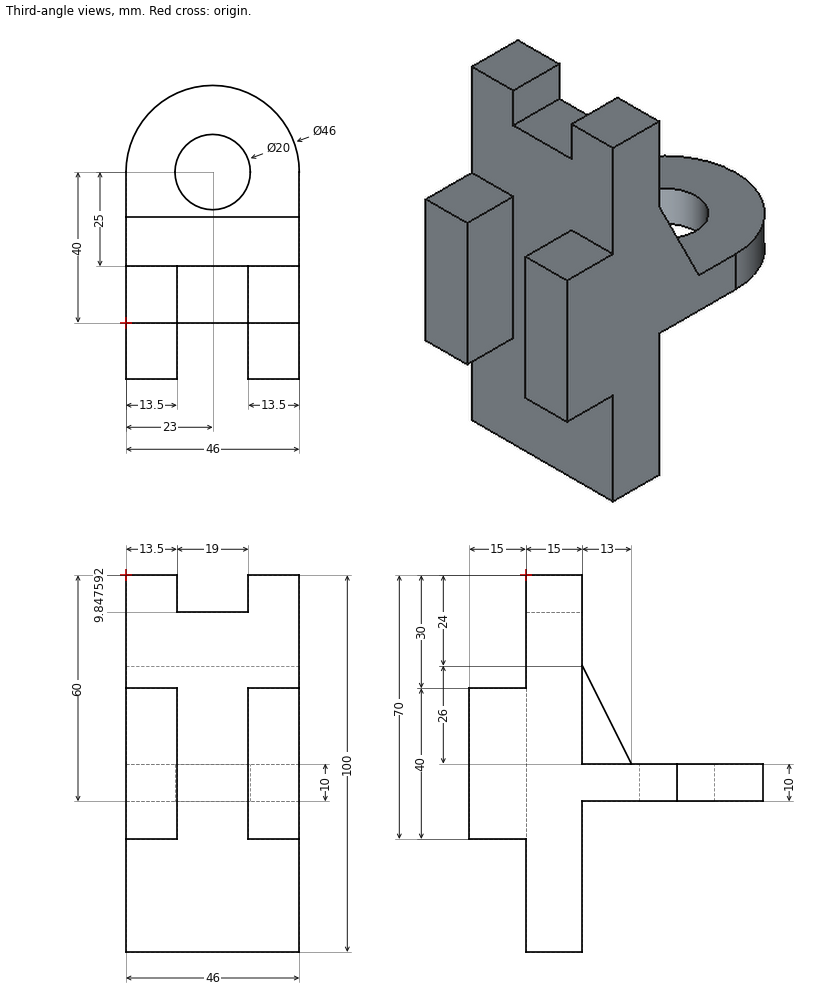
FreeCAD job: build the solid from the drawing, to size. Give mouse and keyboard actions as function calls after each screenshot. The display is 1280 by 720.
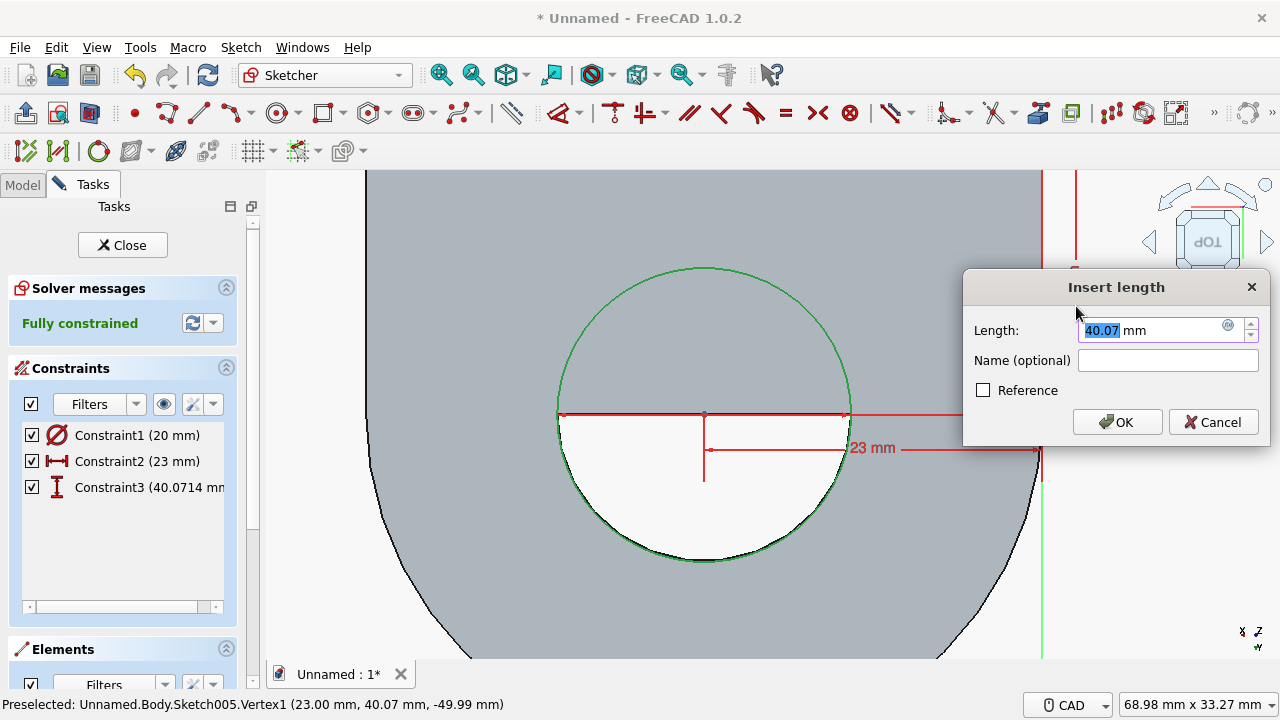
text(40)
key(Return)
key(Escape)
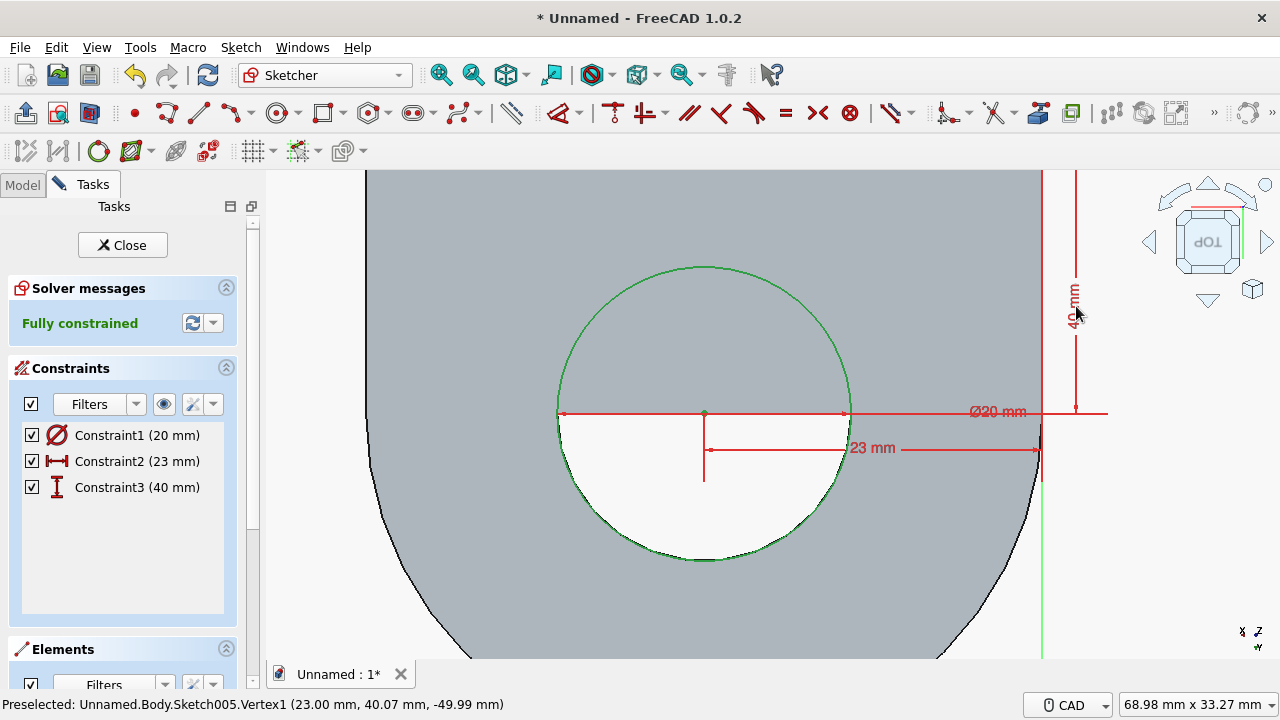
click(123, 245)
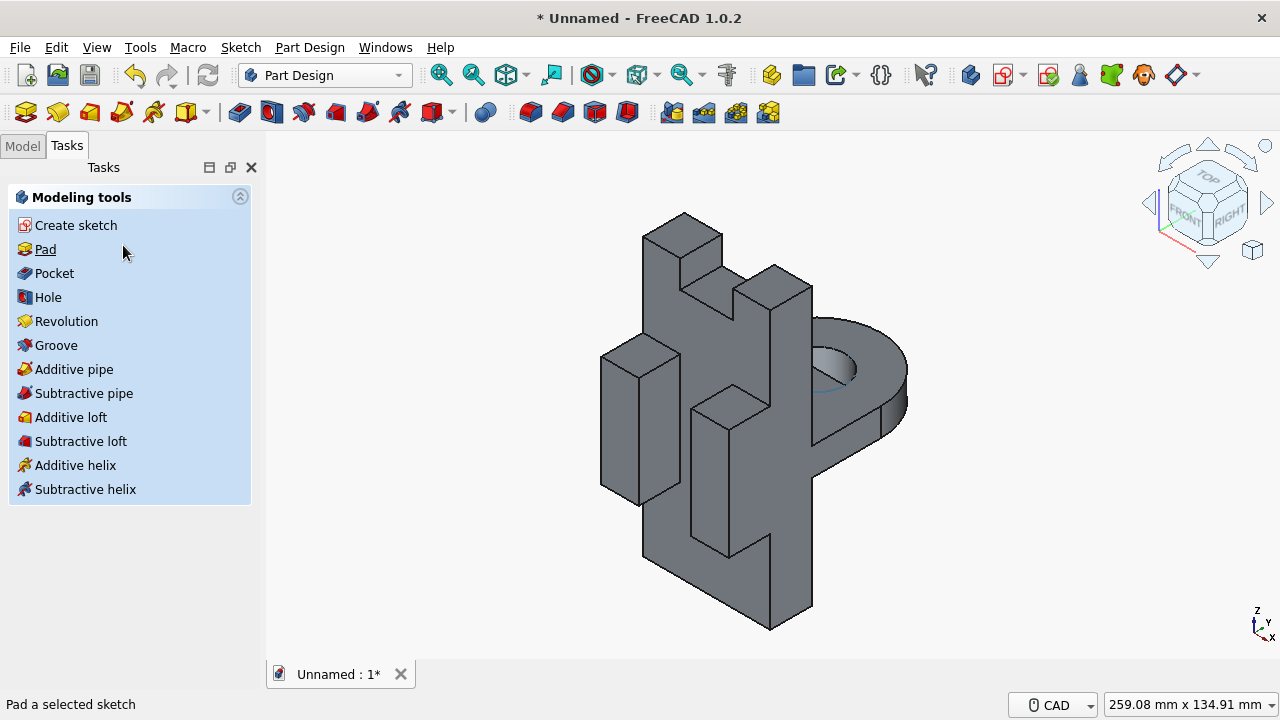
click(240, 112)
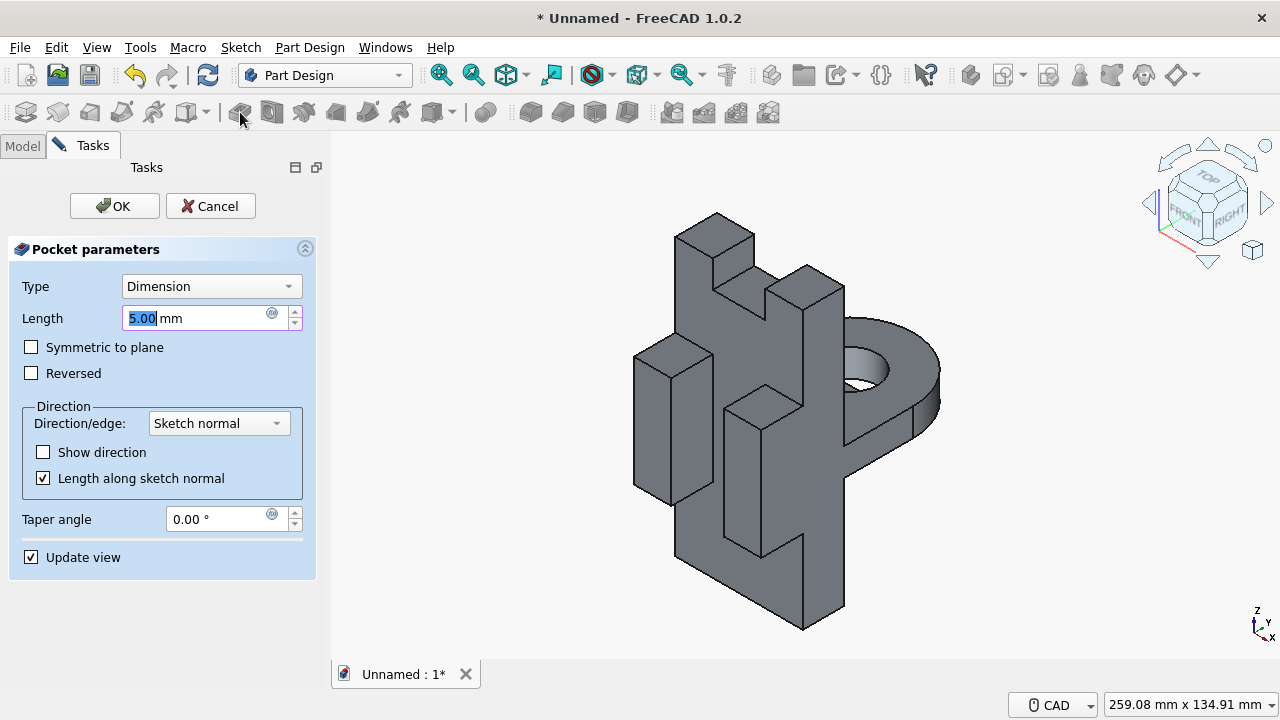
text(10)
key(Tab)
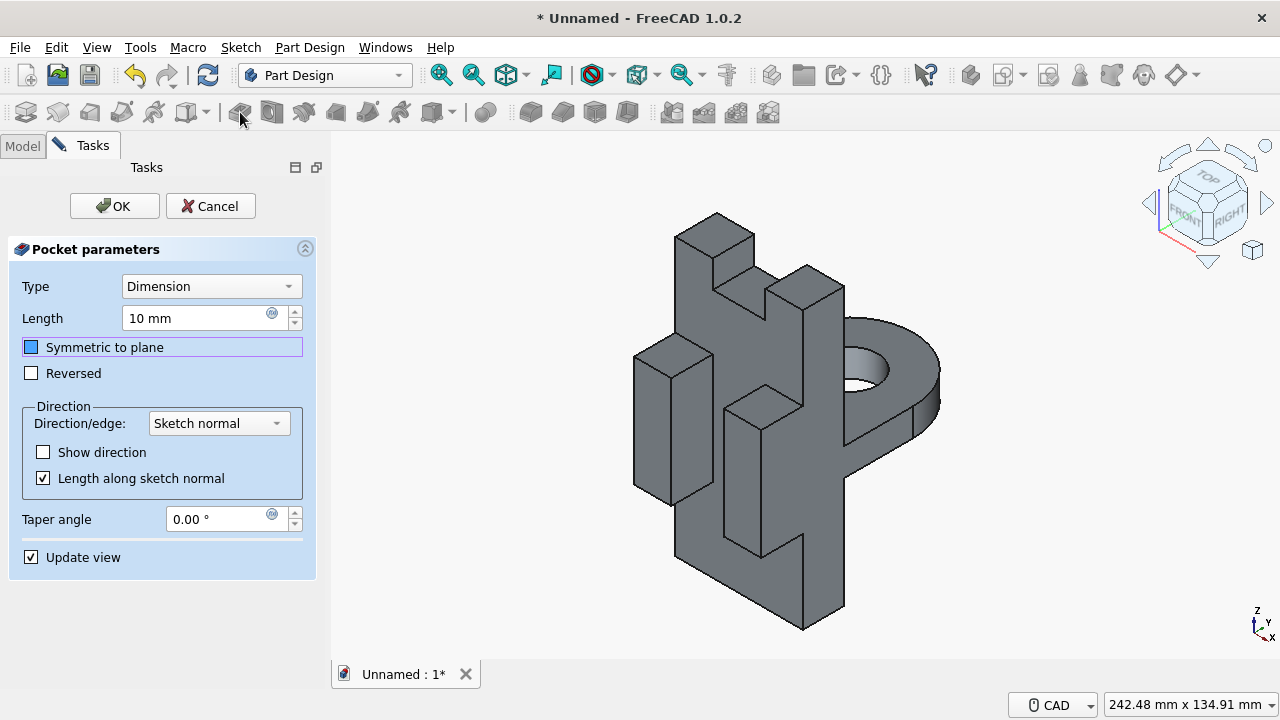
click(115, 206)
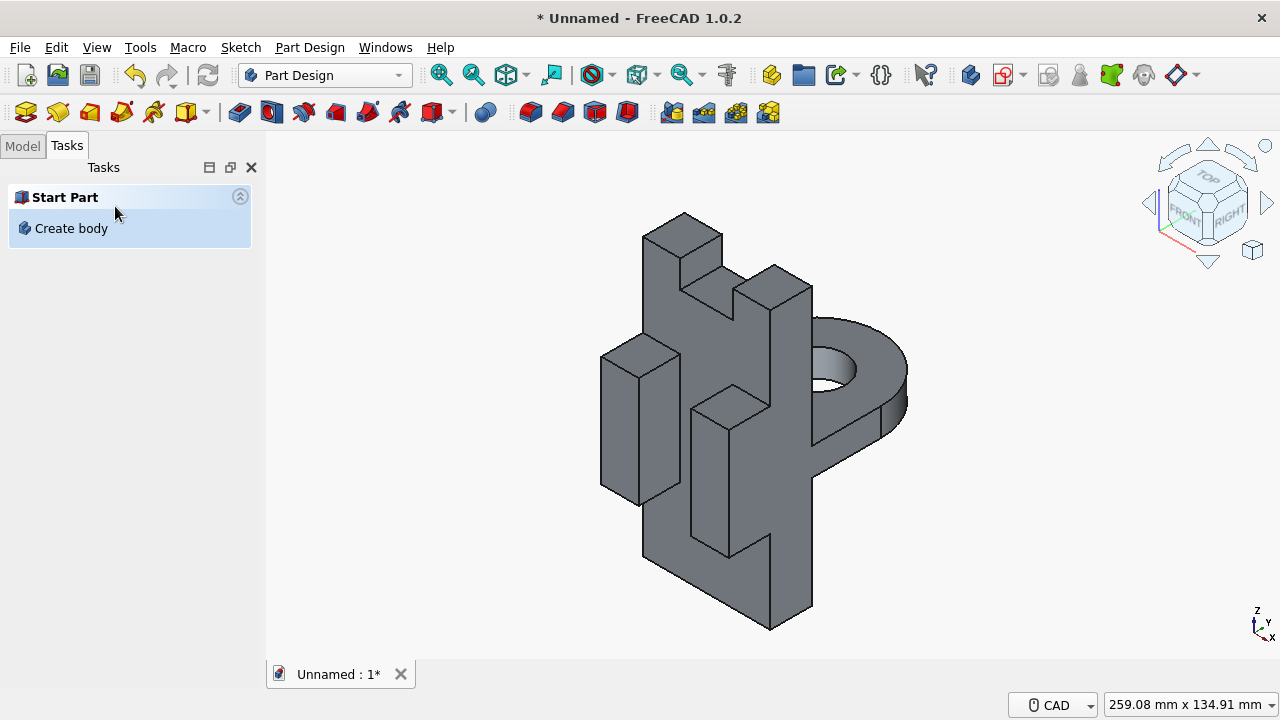
click(761, 474)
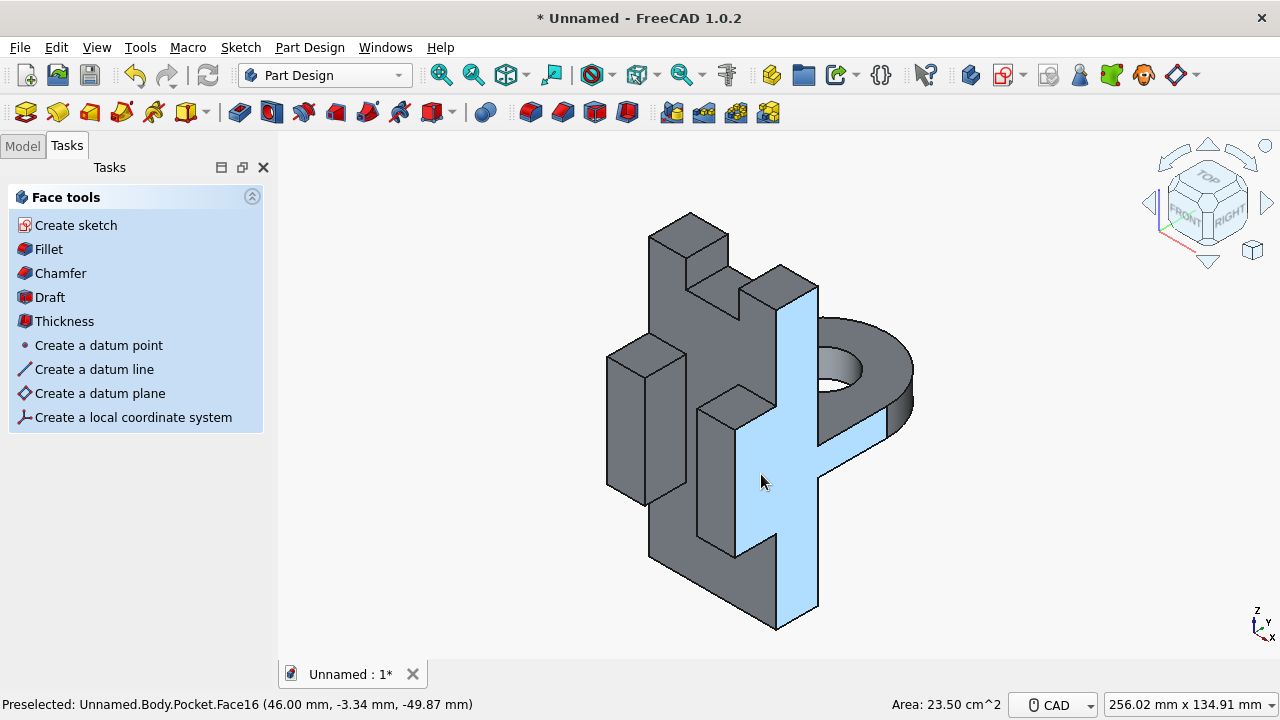
click(1004, 76)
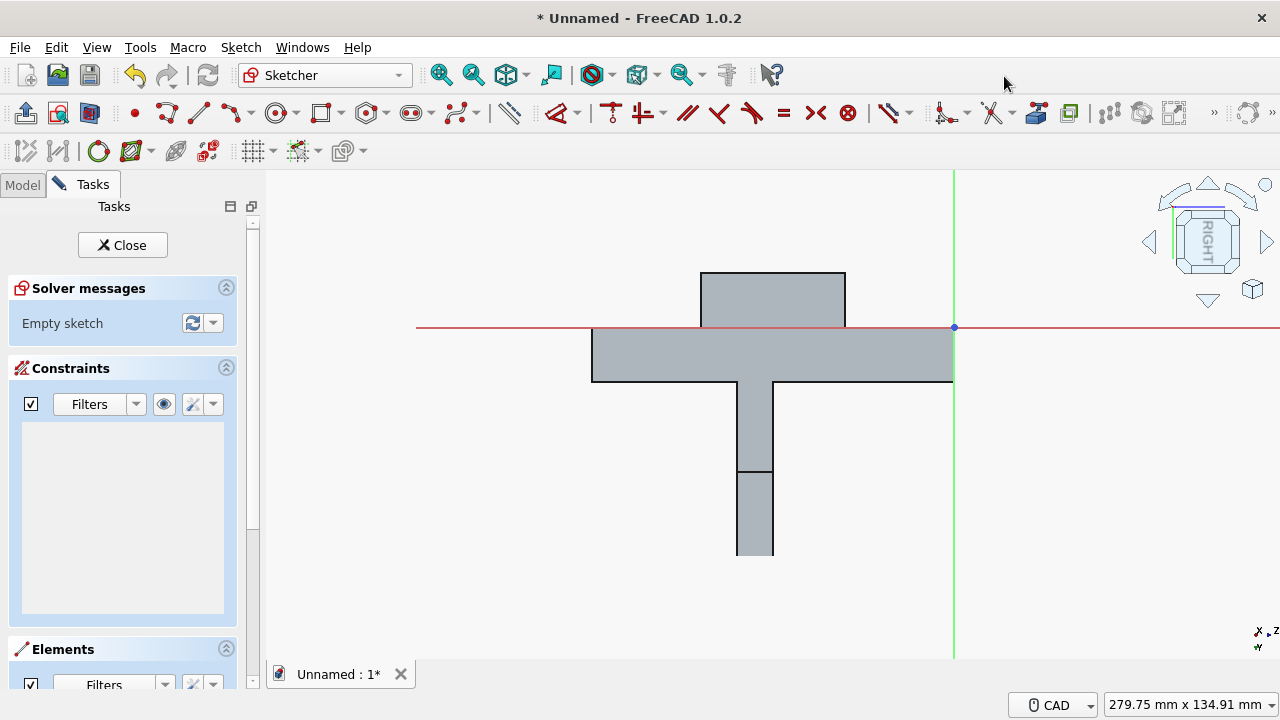
scroll(932, 363, up, 6)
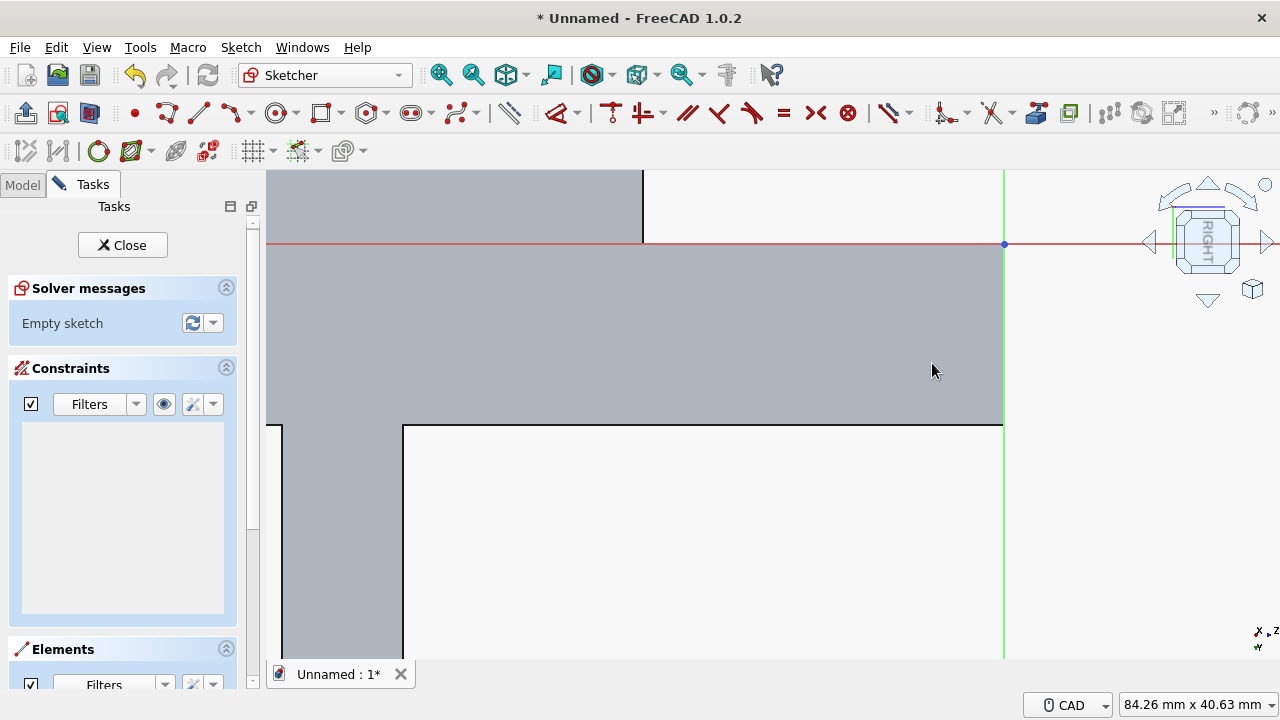
key(g)
key(m)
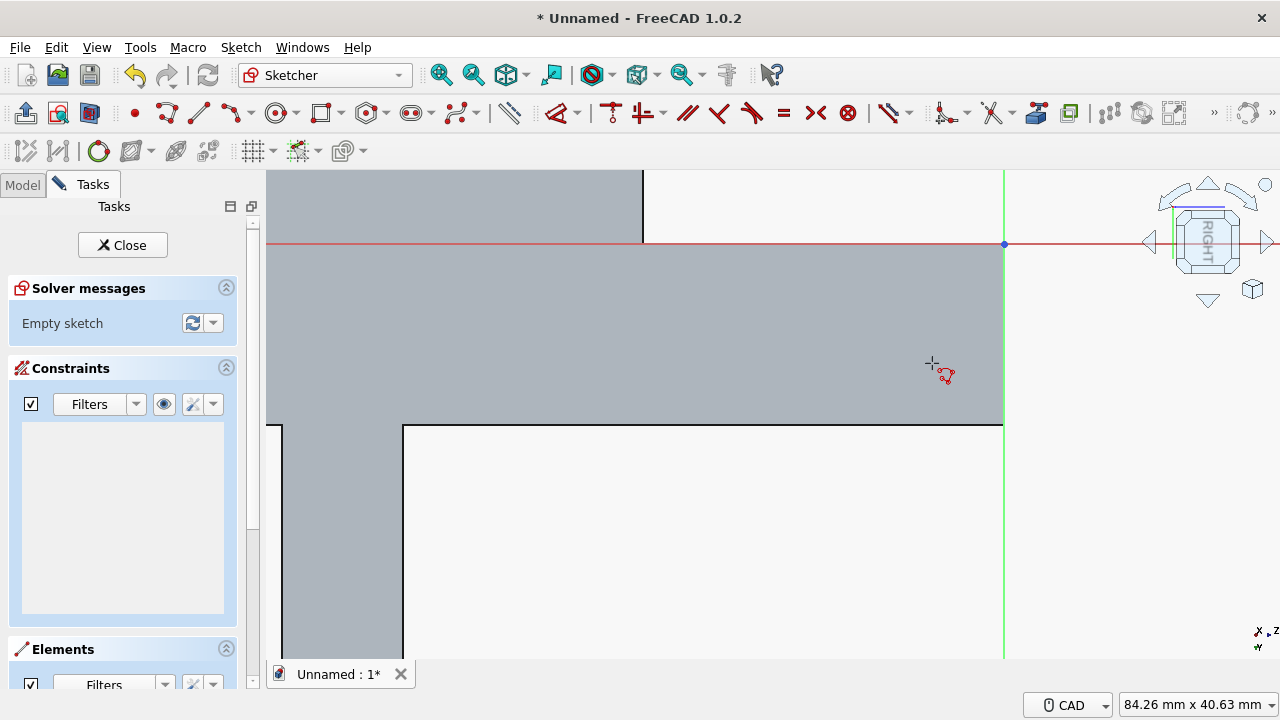
click(715, 425)
click(403, 425)
click(403, 581)
click(715, 426)
key(Escape)
key(Escape)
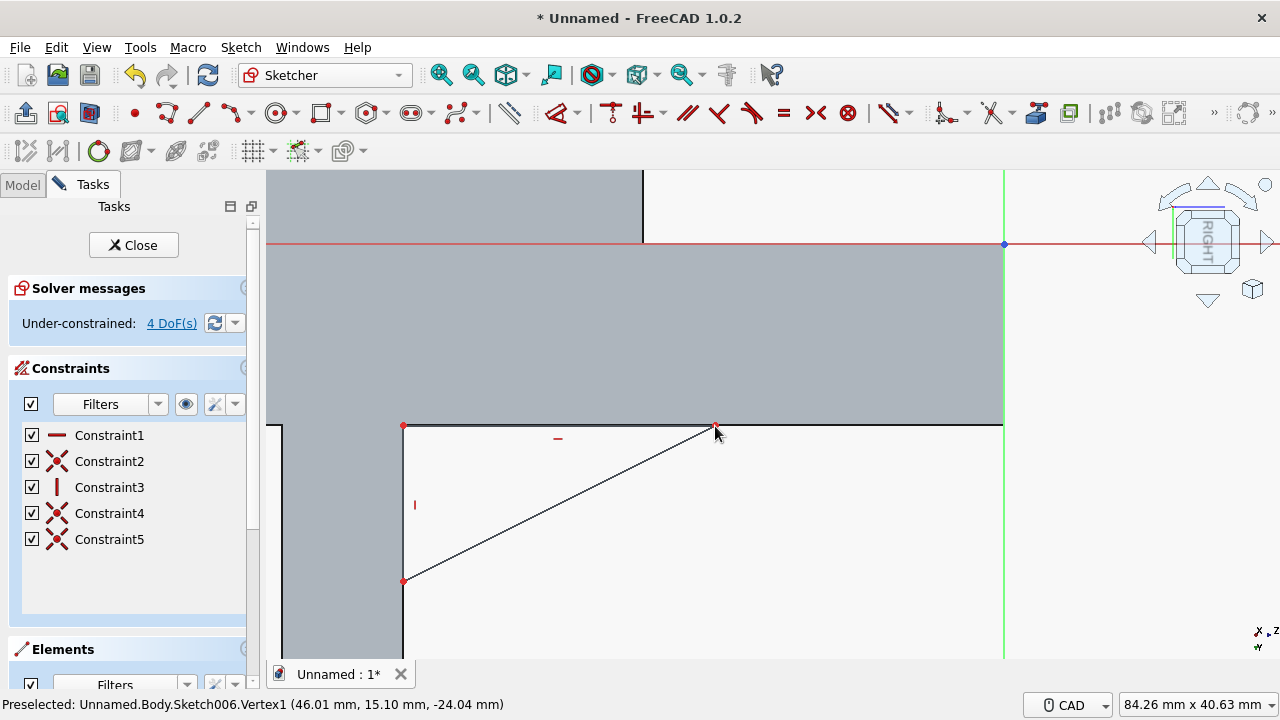
key(d)